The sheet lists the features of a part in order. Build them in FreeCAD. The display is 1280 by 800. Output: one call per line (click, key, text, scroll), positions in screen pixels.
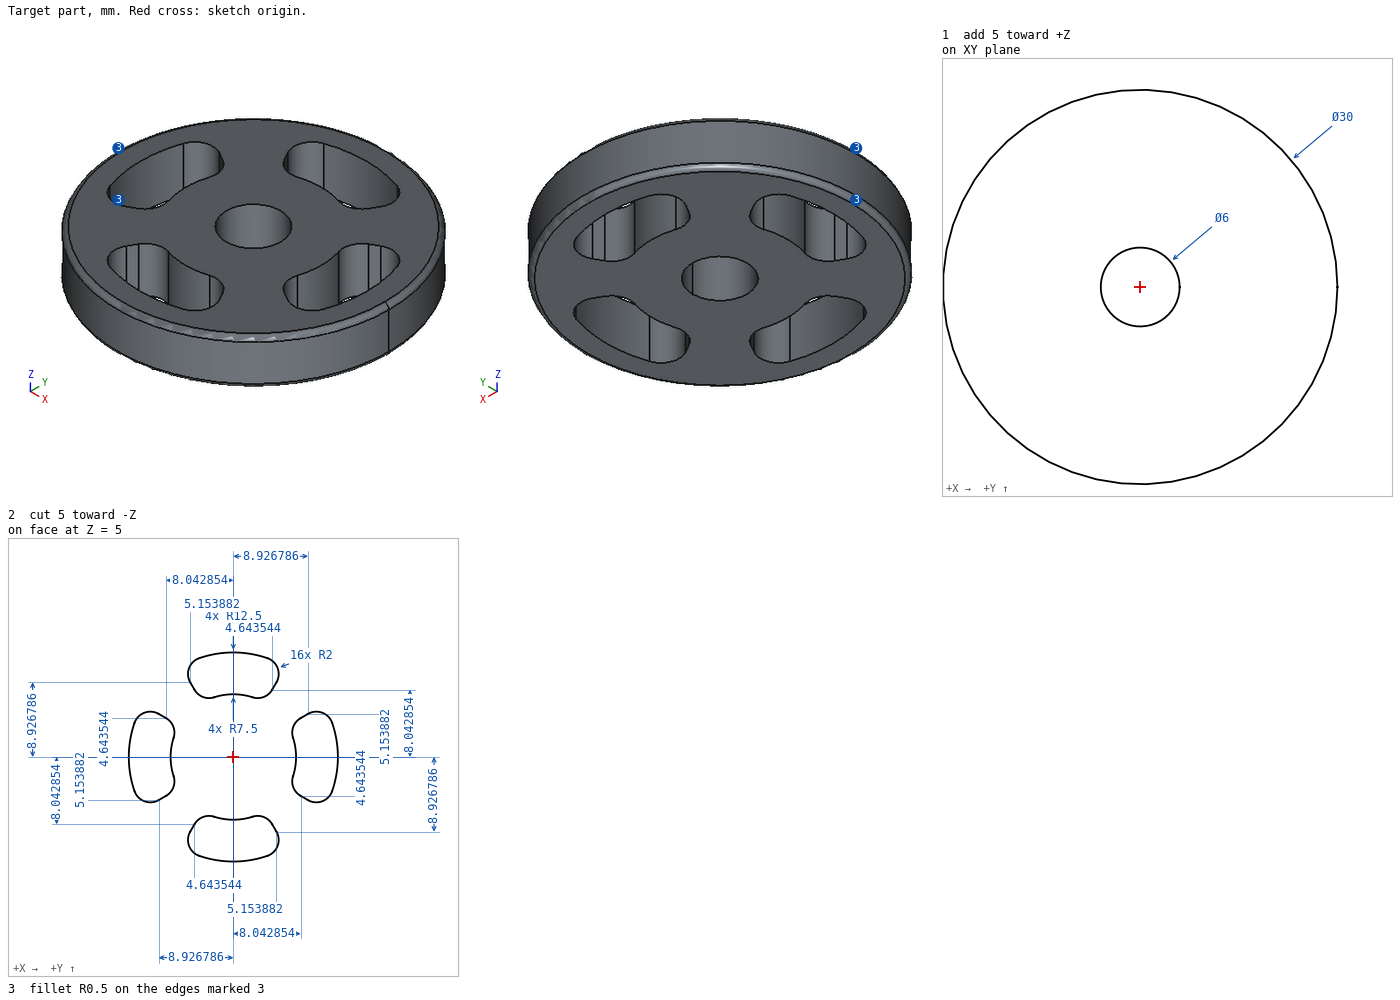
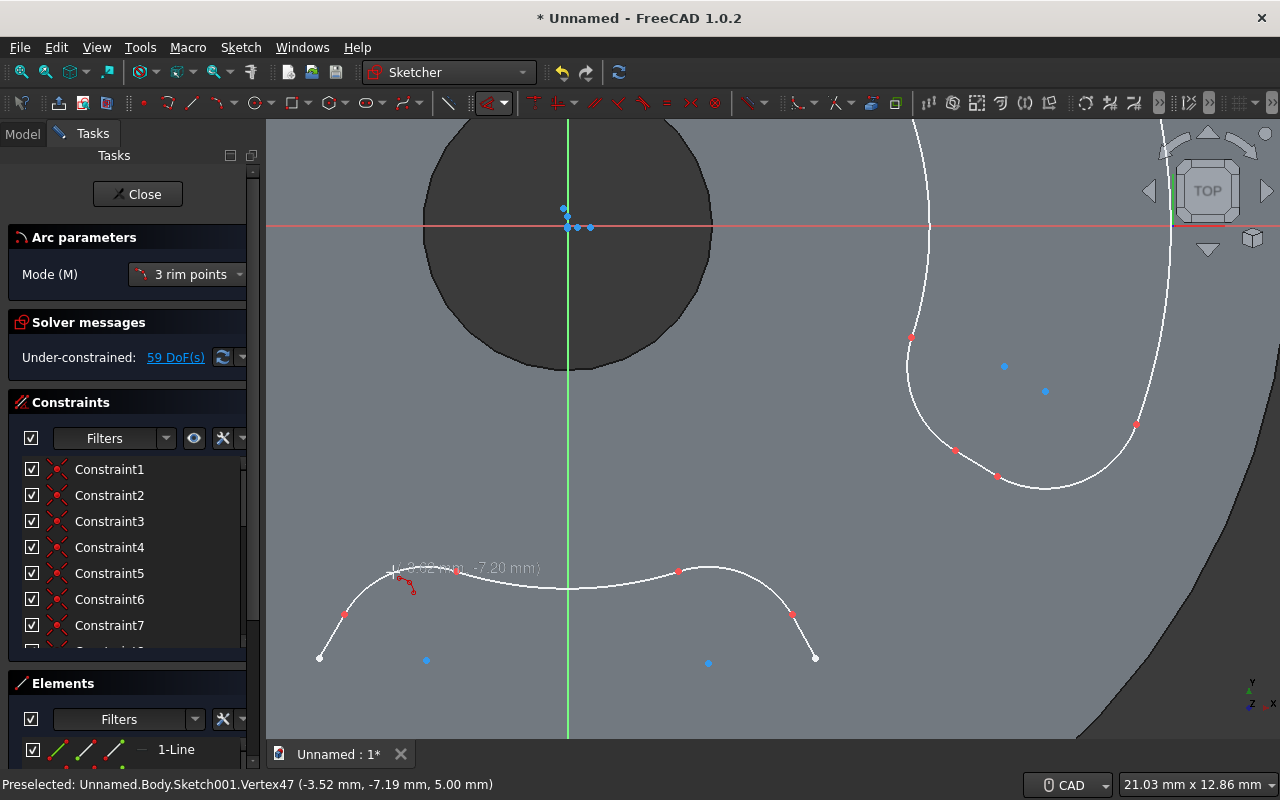
click(319, 658)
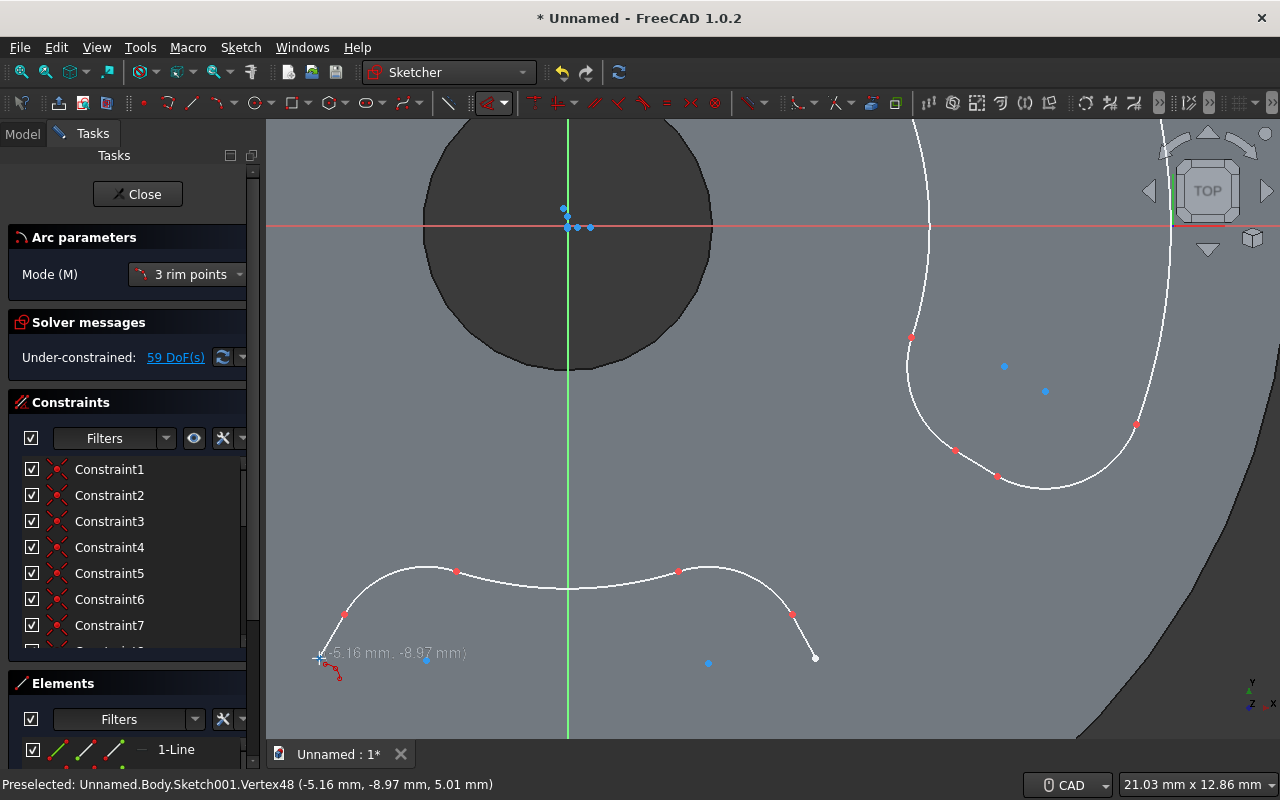
scroll(763, 516, down, 6)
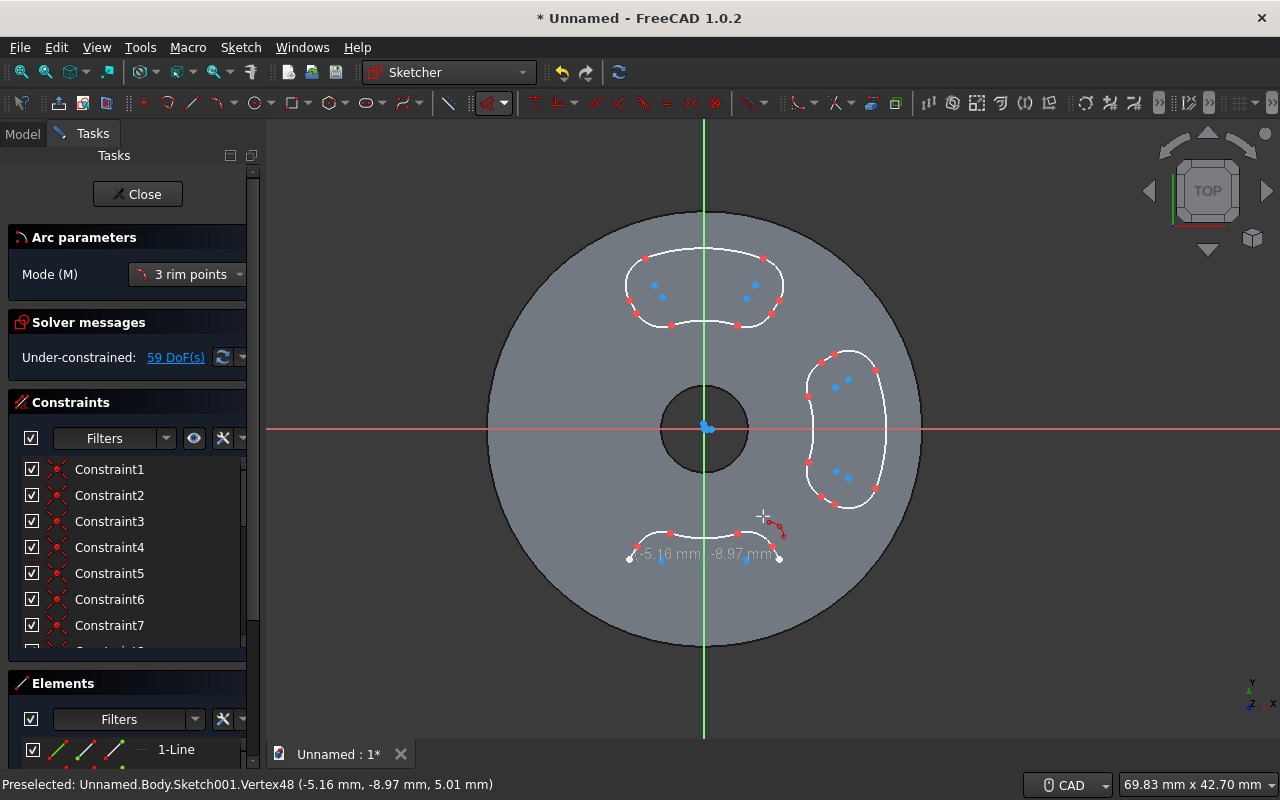
click(645, 601)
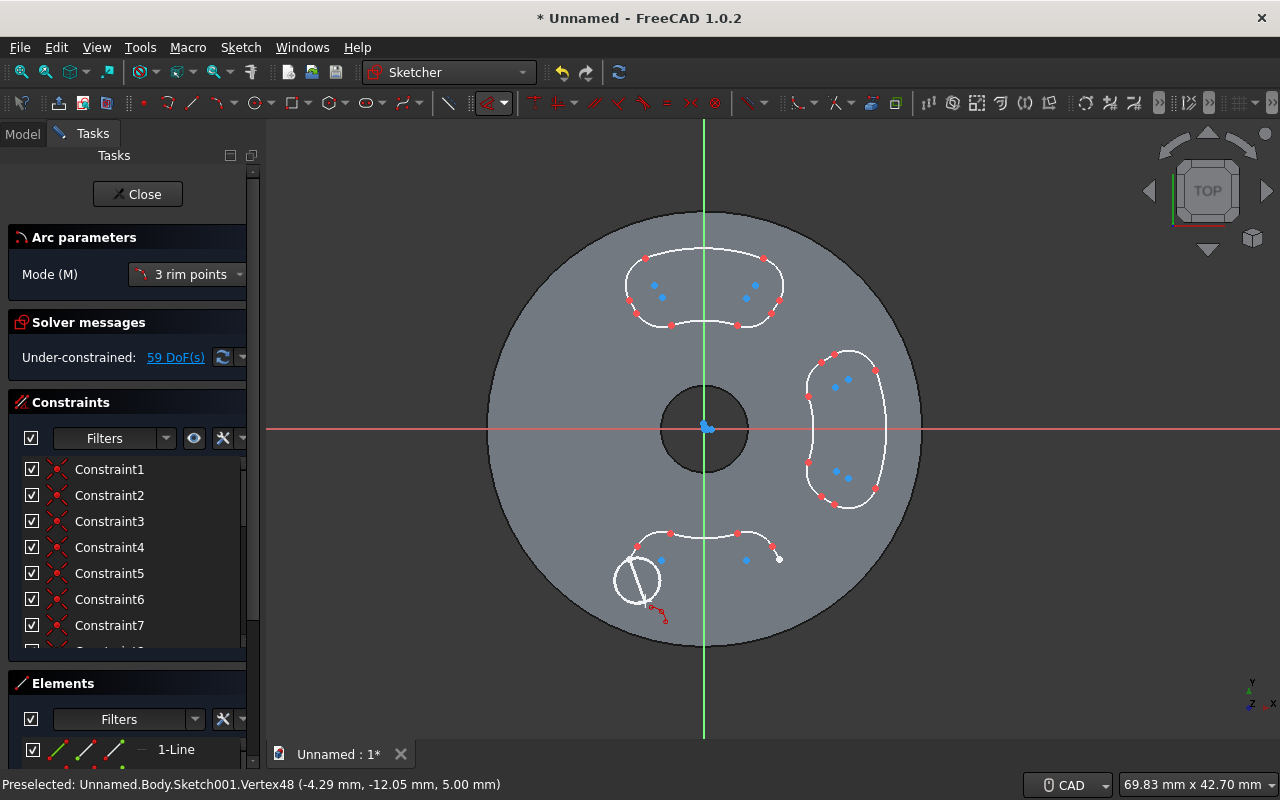
scroll(628, 583, up, 3)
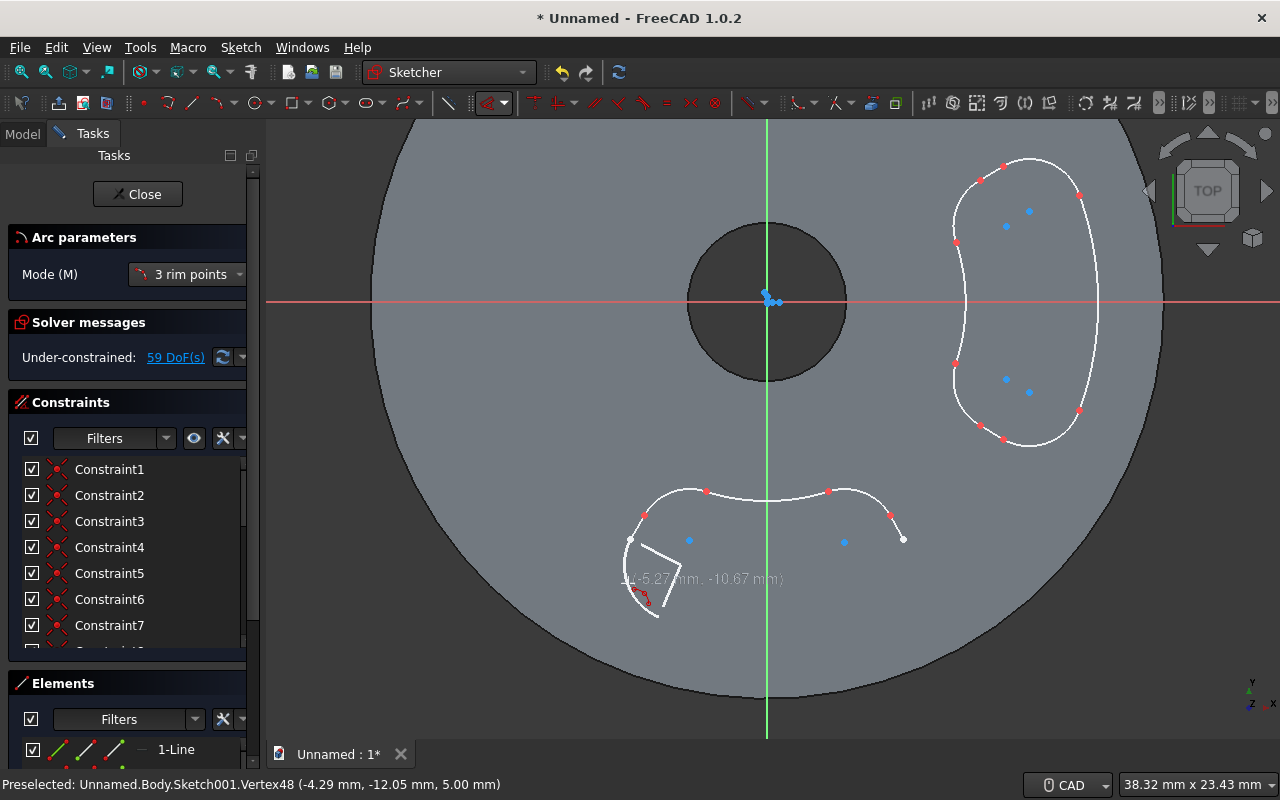
click(627, 583)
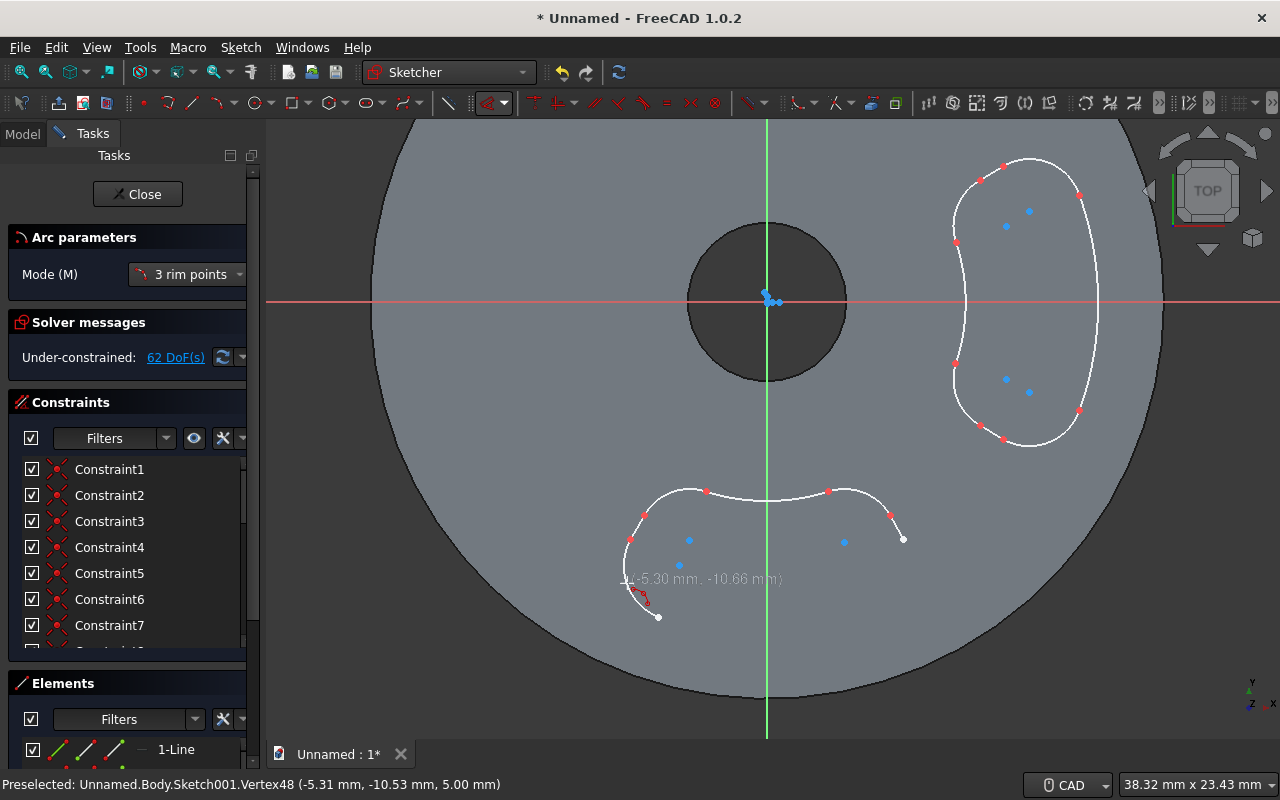
click(659, 617)
click(875, 615)
click(745, 632)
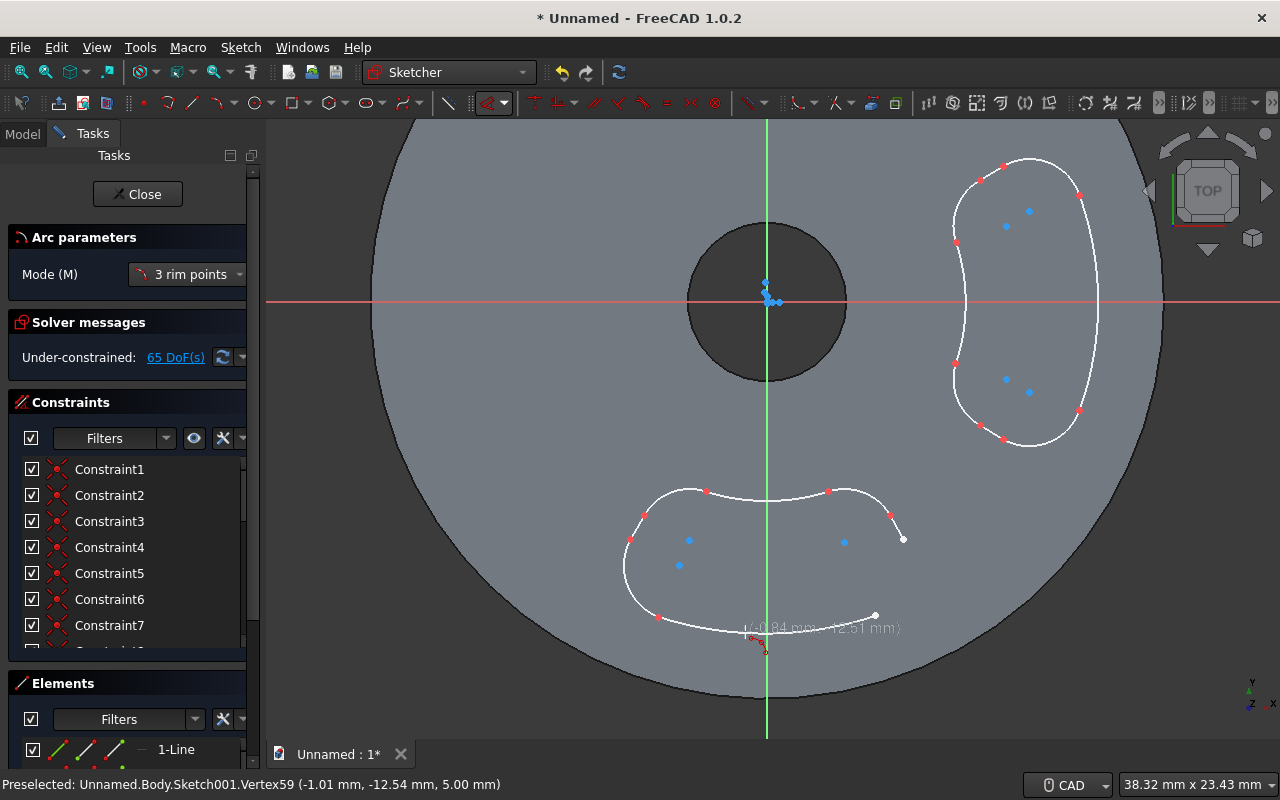
click(875, 616)
click(903, 539)
click(907, 583)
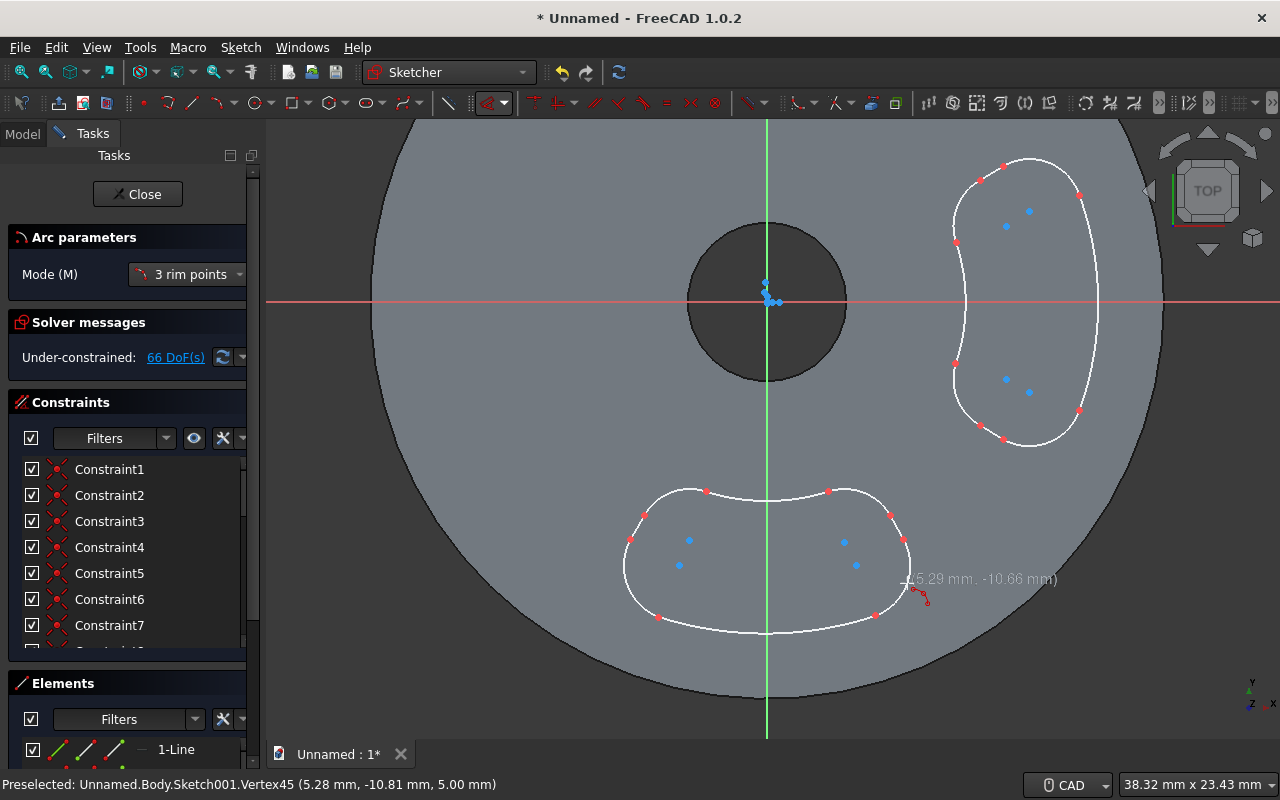
click(192, 104)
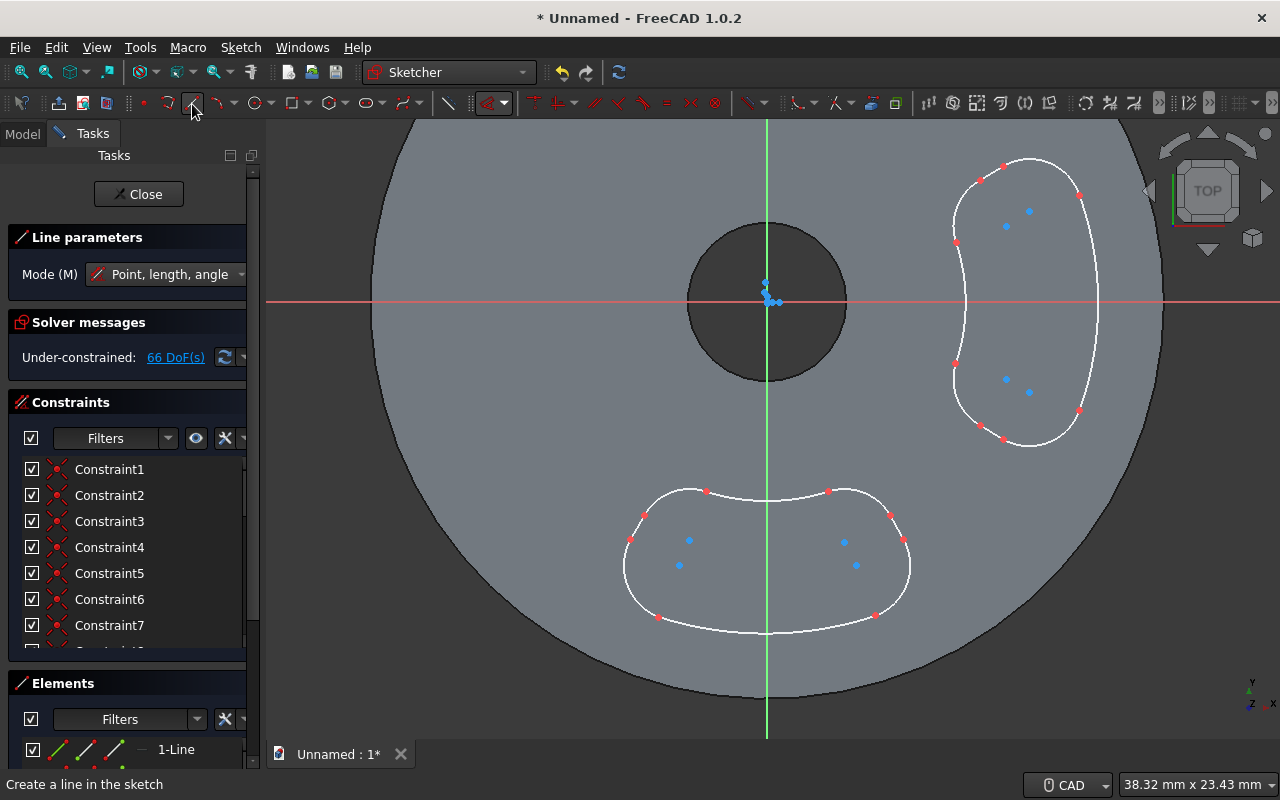
click(531, 438)
click(554, 425)